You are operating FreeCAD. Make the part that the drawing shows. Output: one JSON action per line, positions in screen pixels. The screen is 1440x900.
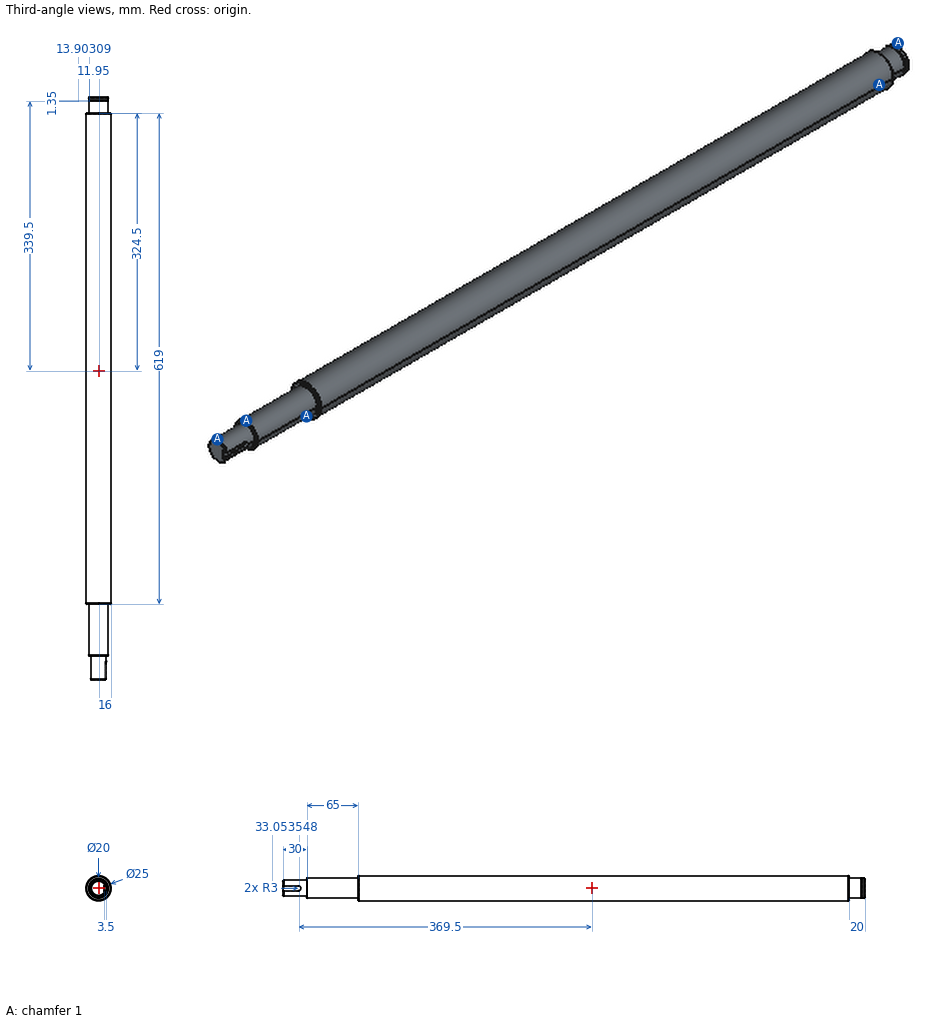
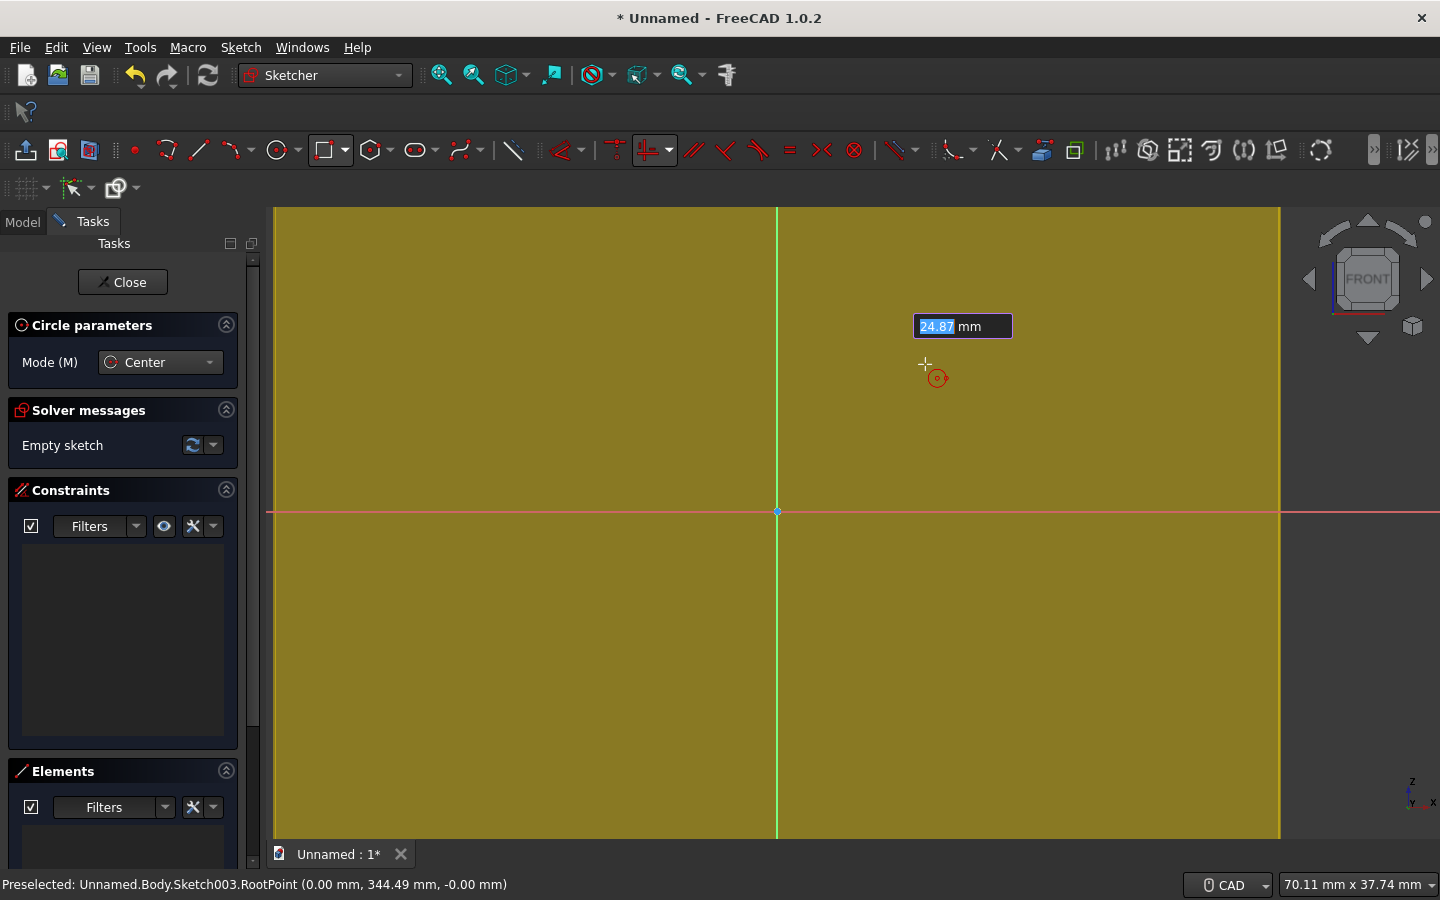
{"action": "type", "text": "25"}
{"action": "key", "text": "Return"}
{"action": "key", "text": "Escape"}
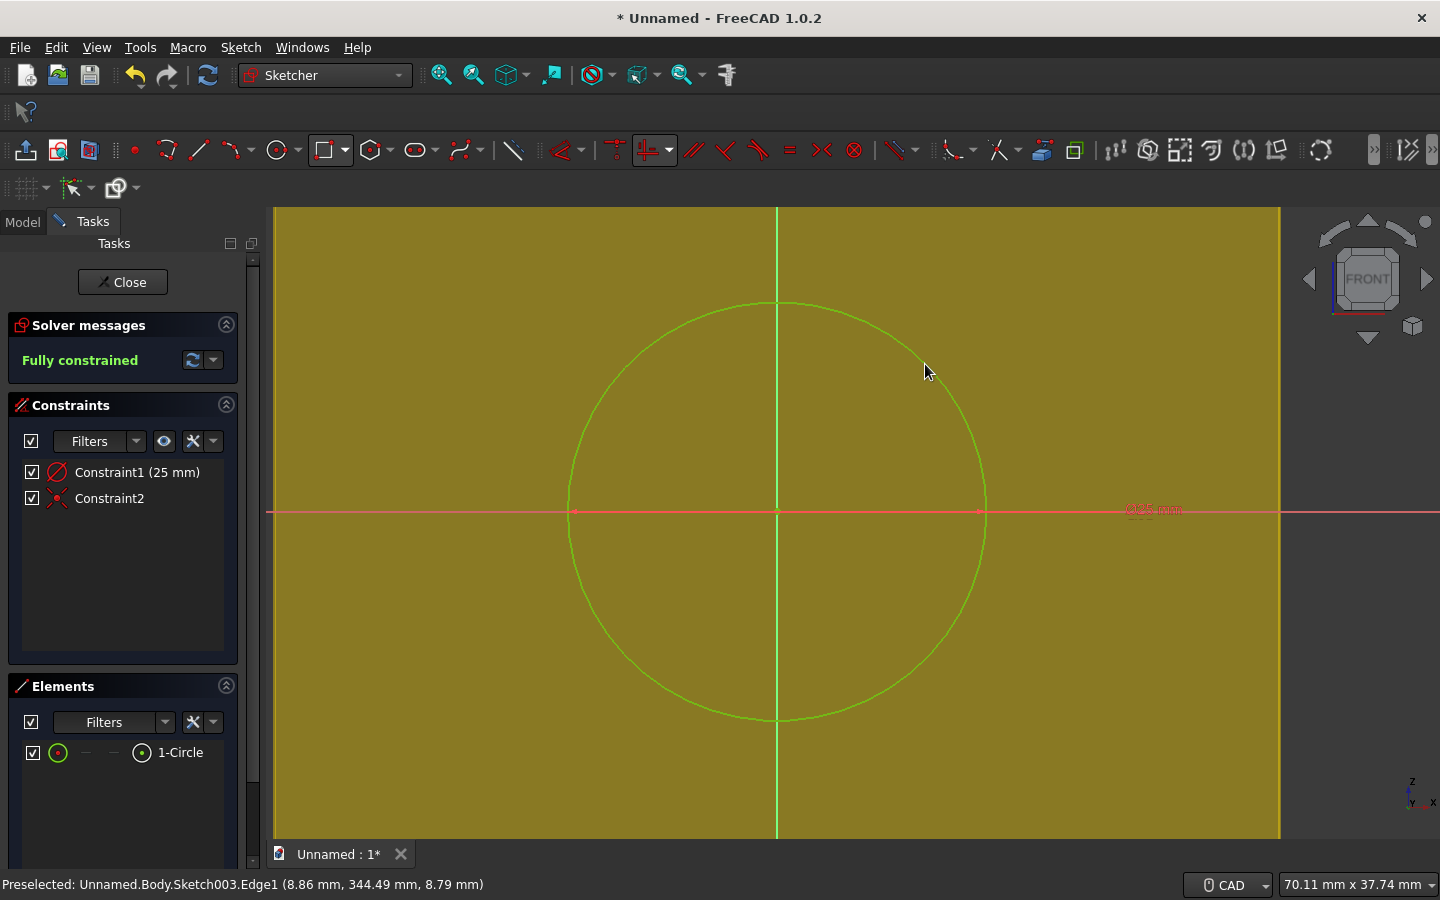
{"action": "left_click", "coordinate": [123, 282]}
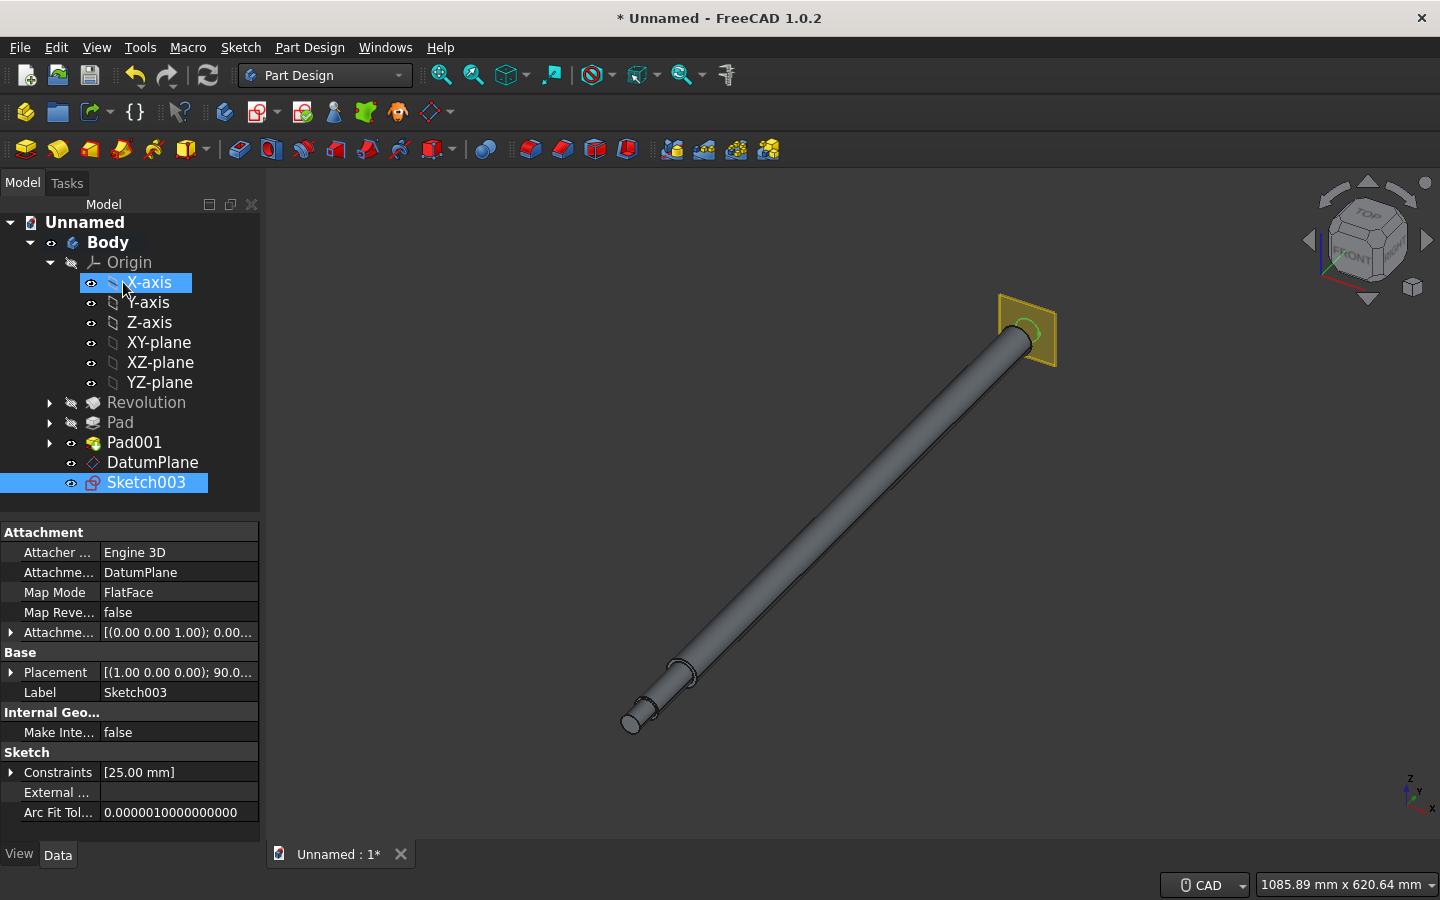
{"action": "left_click", "coordinate": [26, 150]}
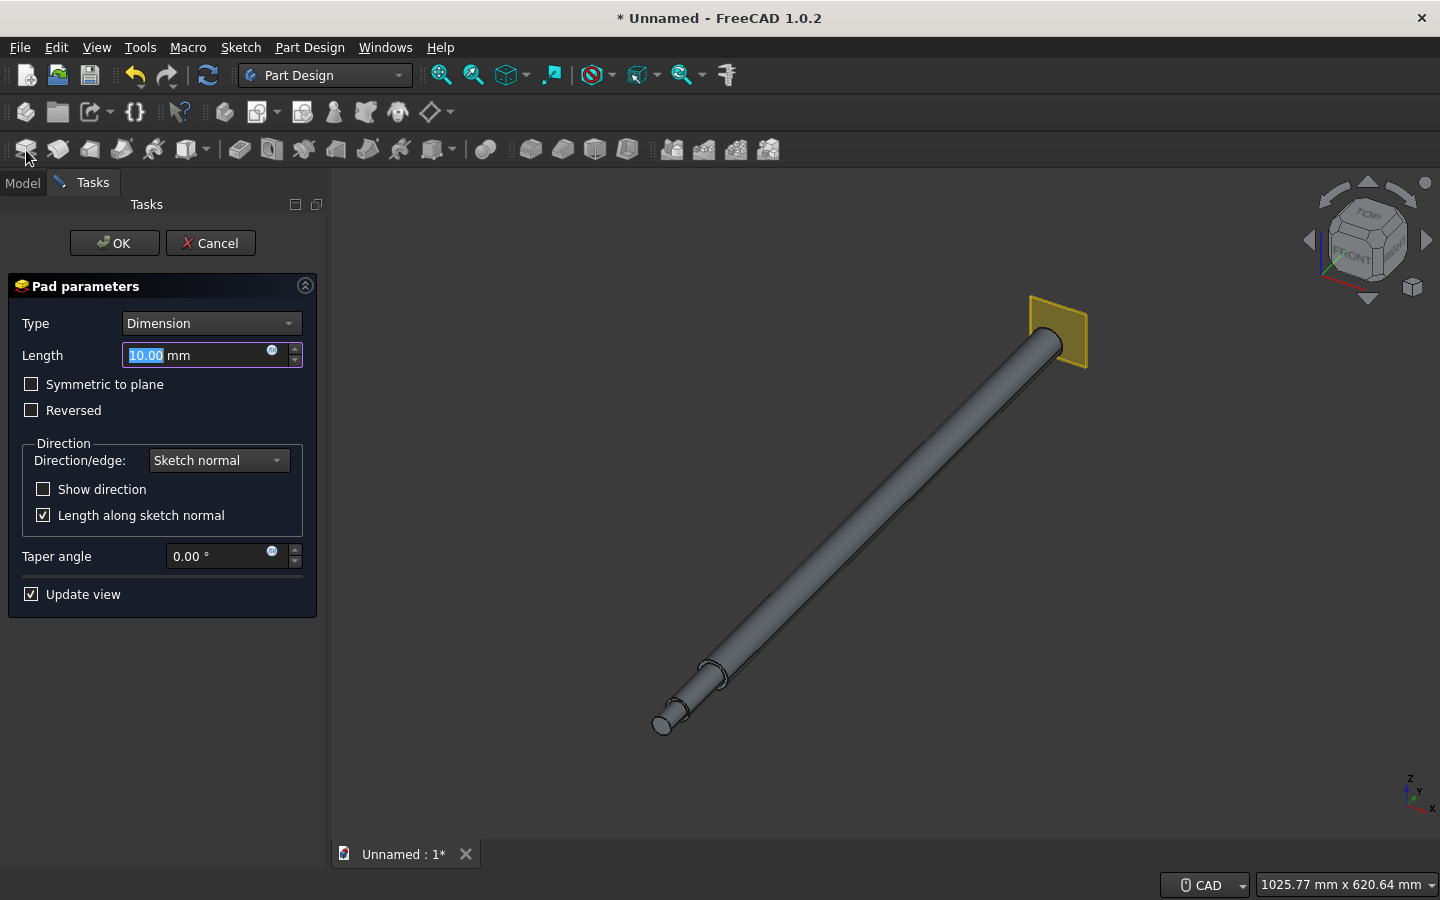
{"action": "type", "text": "20"}
{"action": "key", "text": "Tab"}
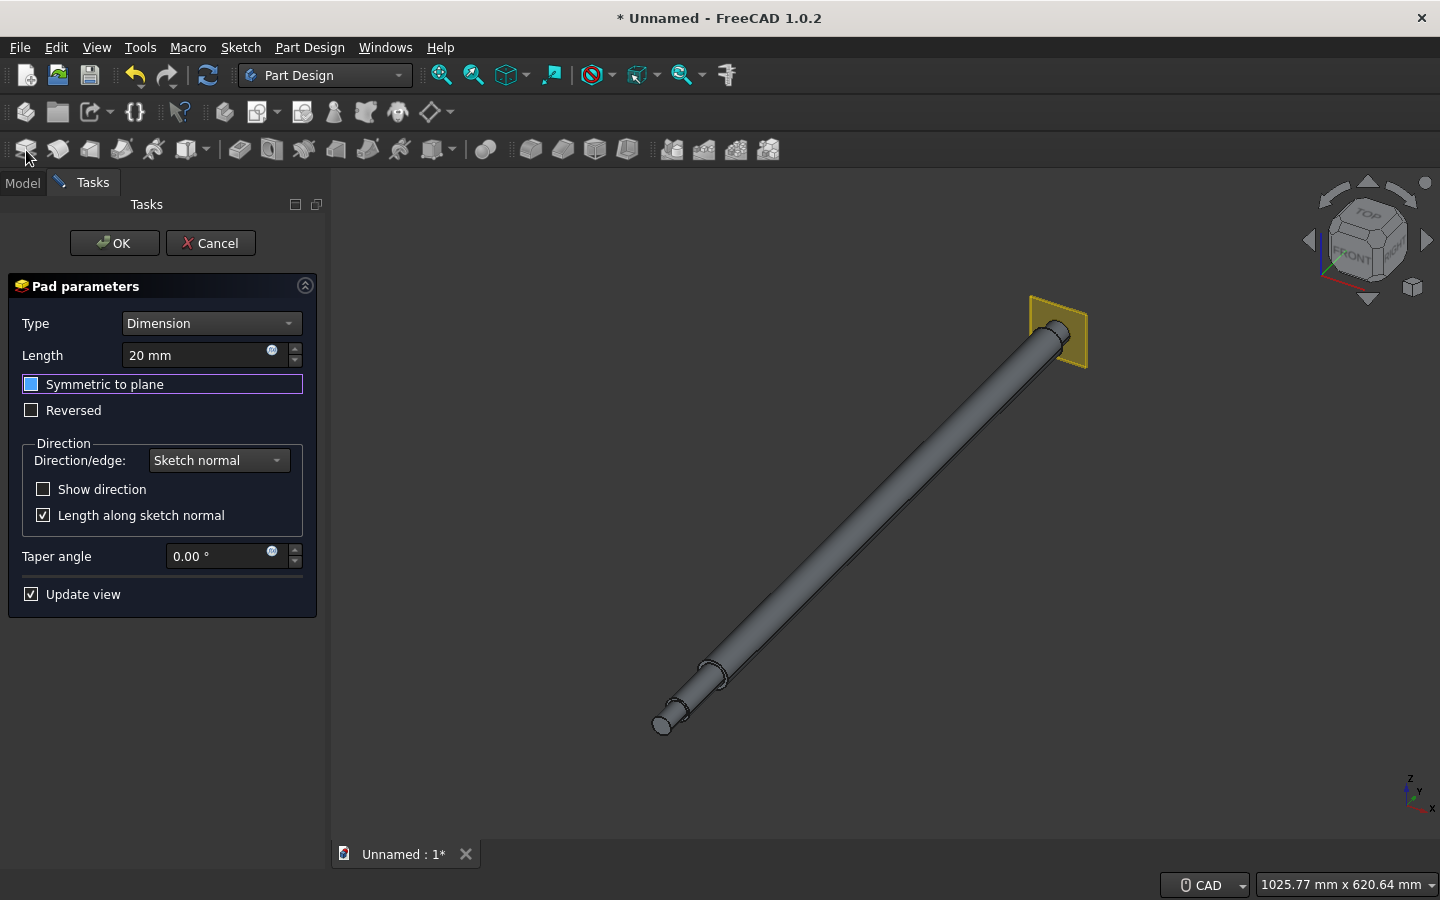
{"action": "left_click", "coordinate": [115, 243]}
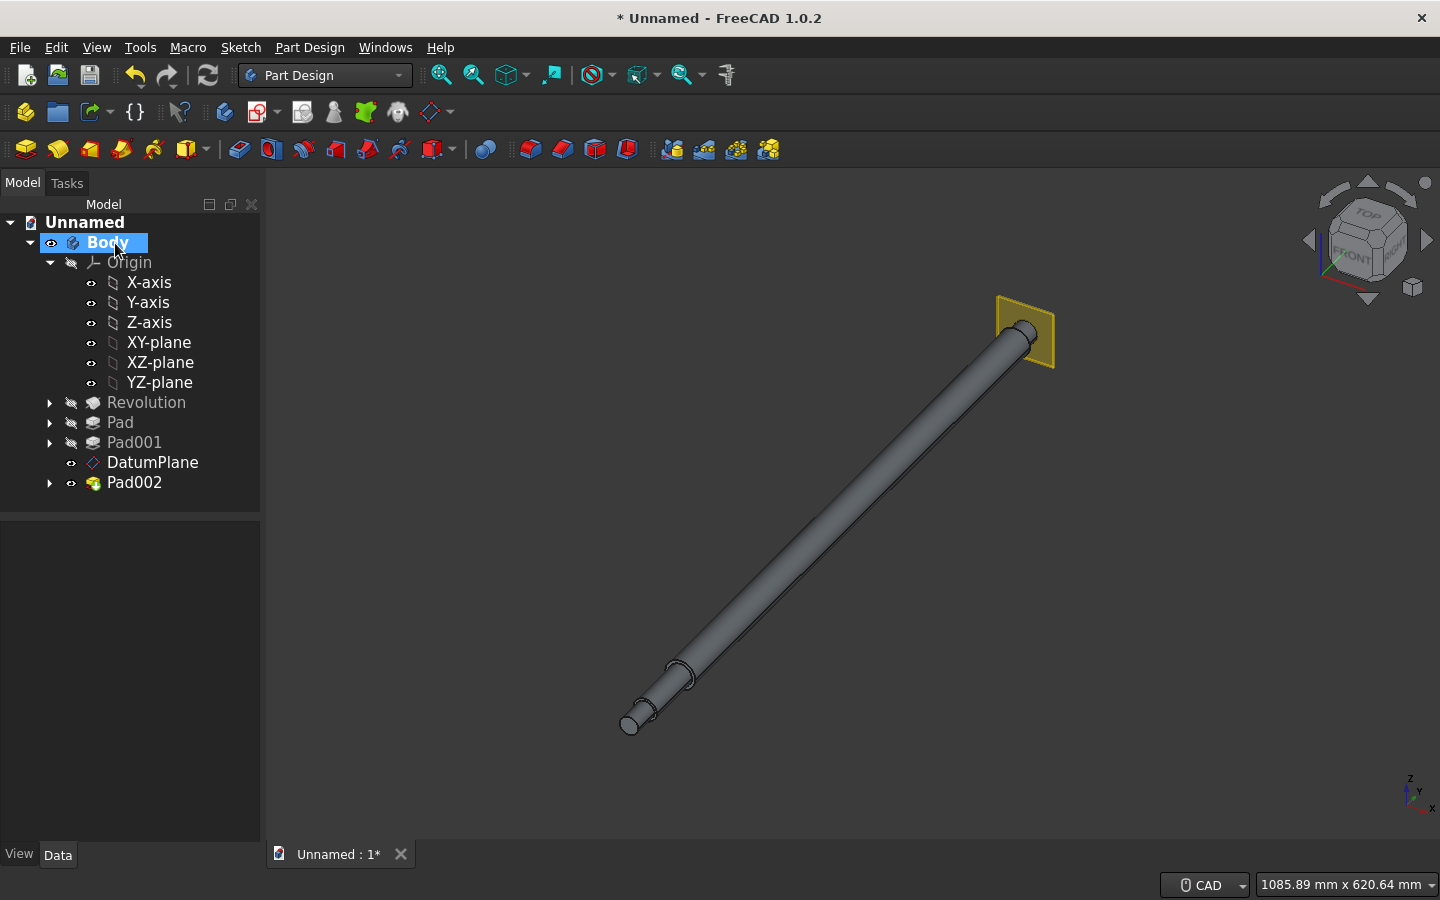
{"action": "left_click", "coordinate": [116, 463]}
{"action": "key", "text": "space"}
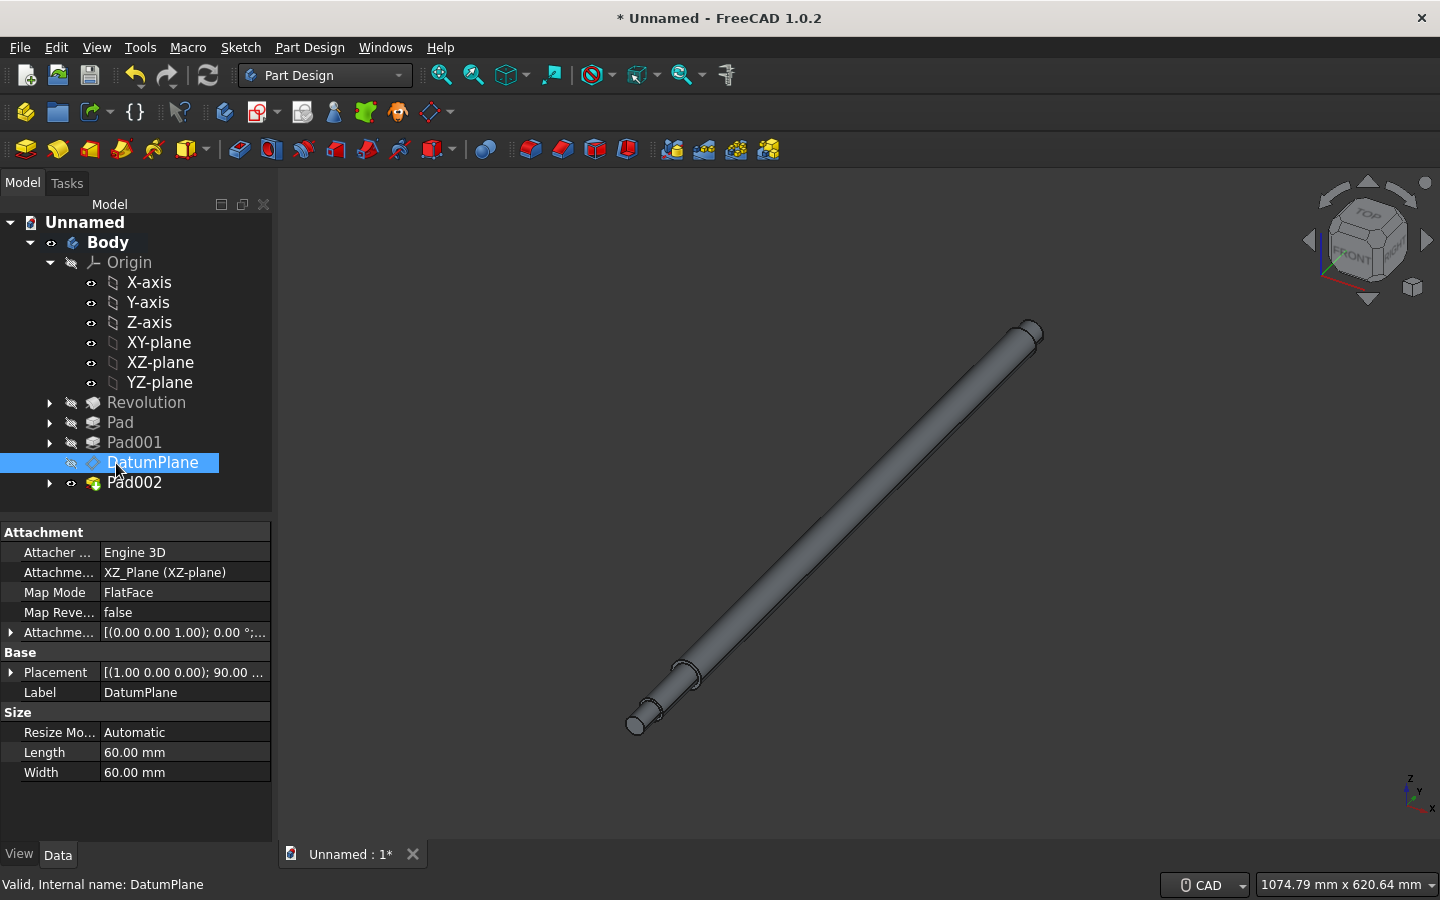
{"action": "left_click", "coordinate": [318, 799]}